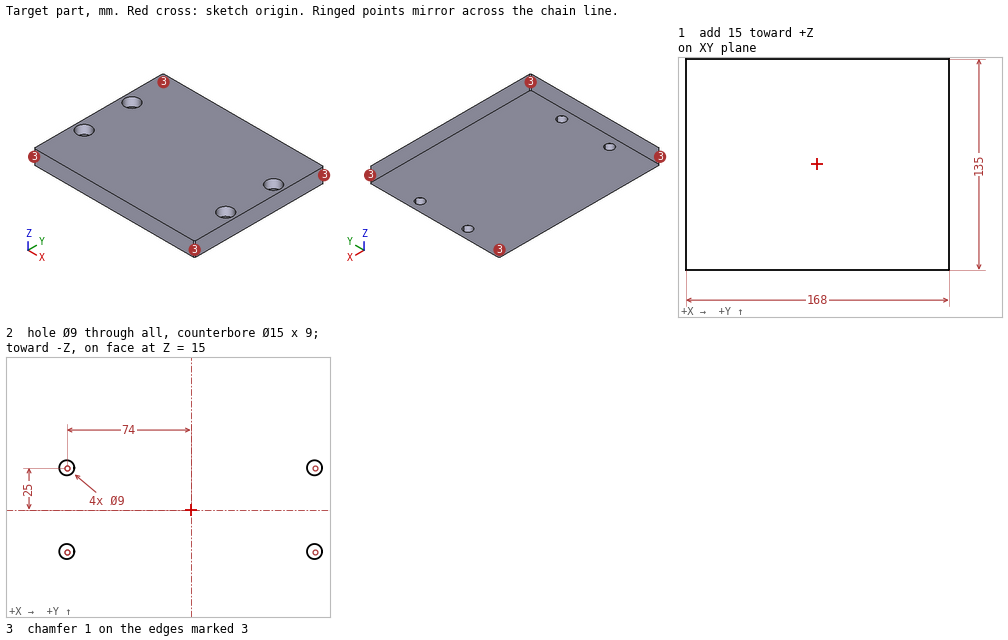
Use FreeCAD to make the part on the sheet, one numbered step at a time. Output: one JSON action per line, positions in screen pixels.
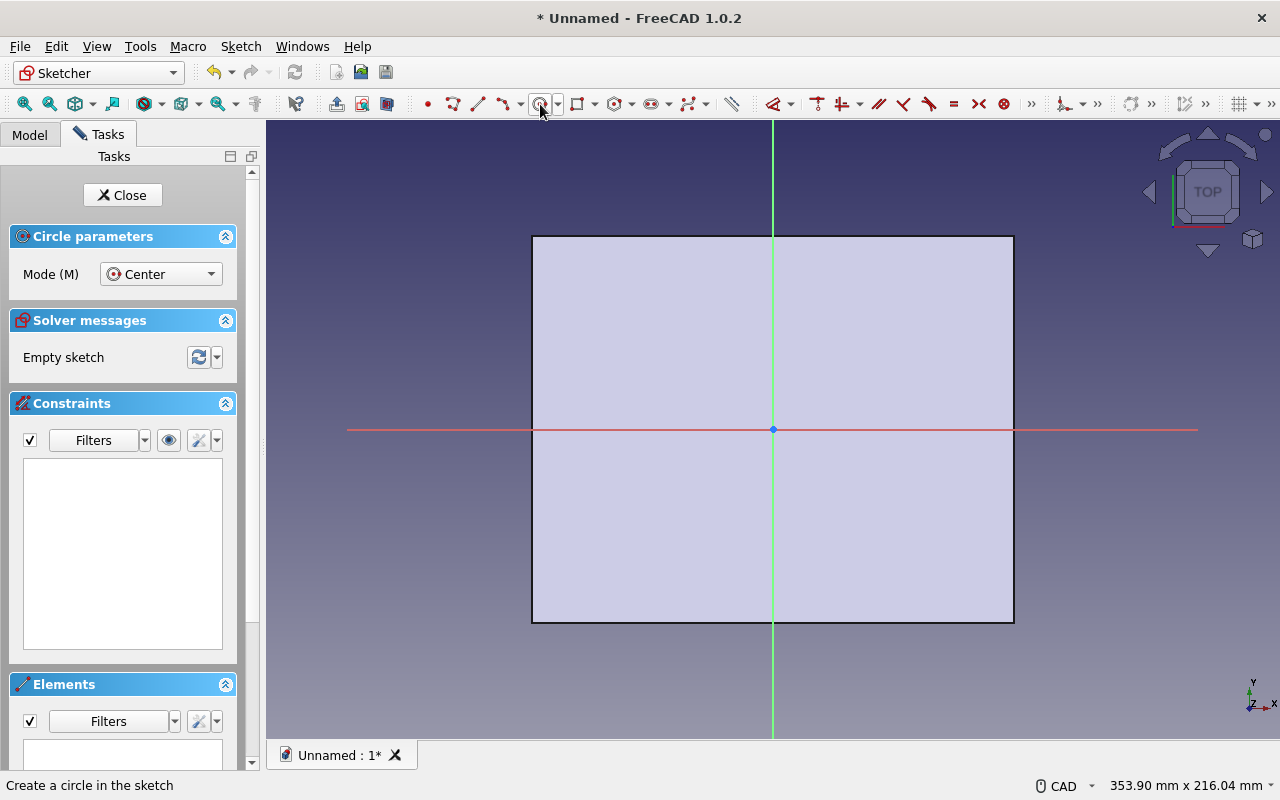
{"action": "scroll", "coordinate": [561, 358], "scroll_direction": "up", "scroll_amount": 3}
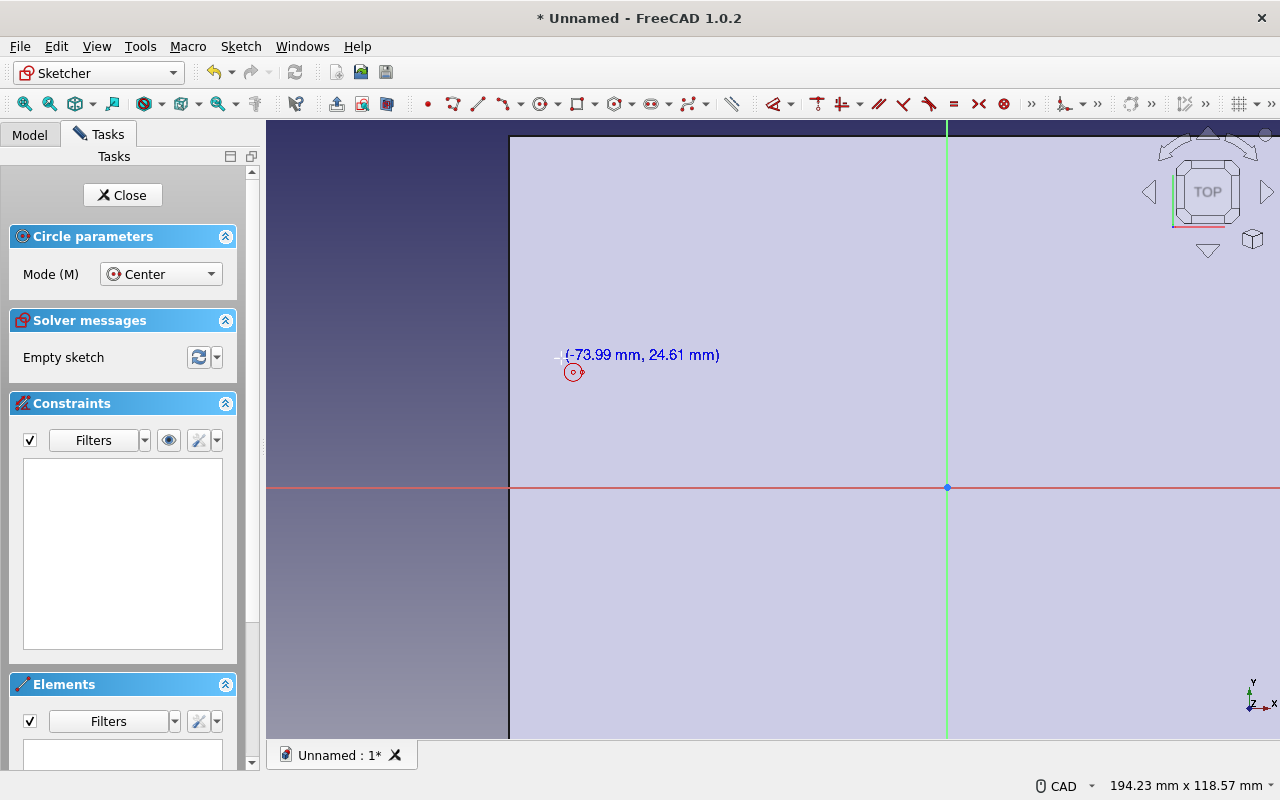
{"action": "left_click", "coordinate": [561, 357]}
{"action": "left_click", "coordinate": [577, 341]}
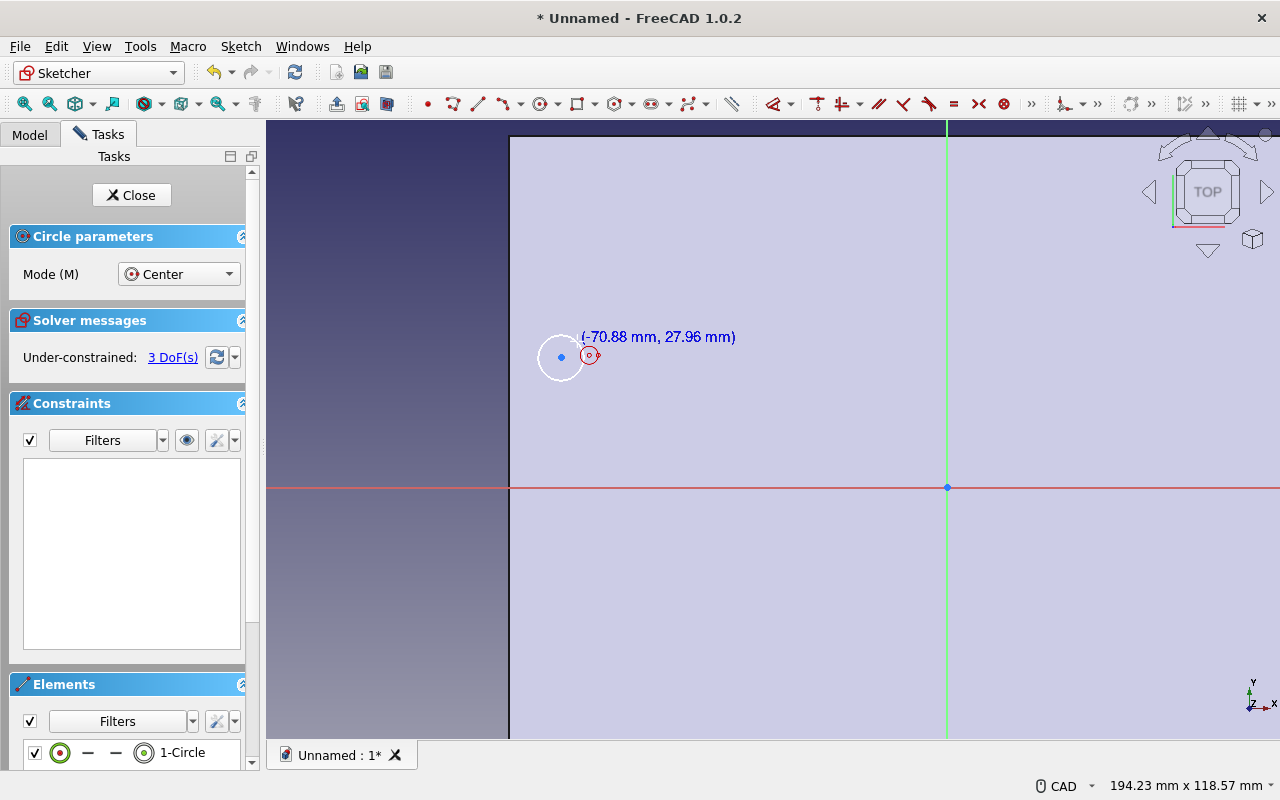
{"action": "left_click", "coordinate": [561, 618]}
{"action": "left_click", "coordinate": [577, 602]}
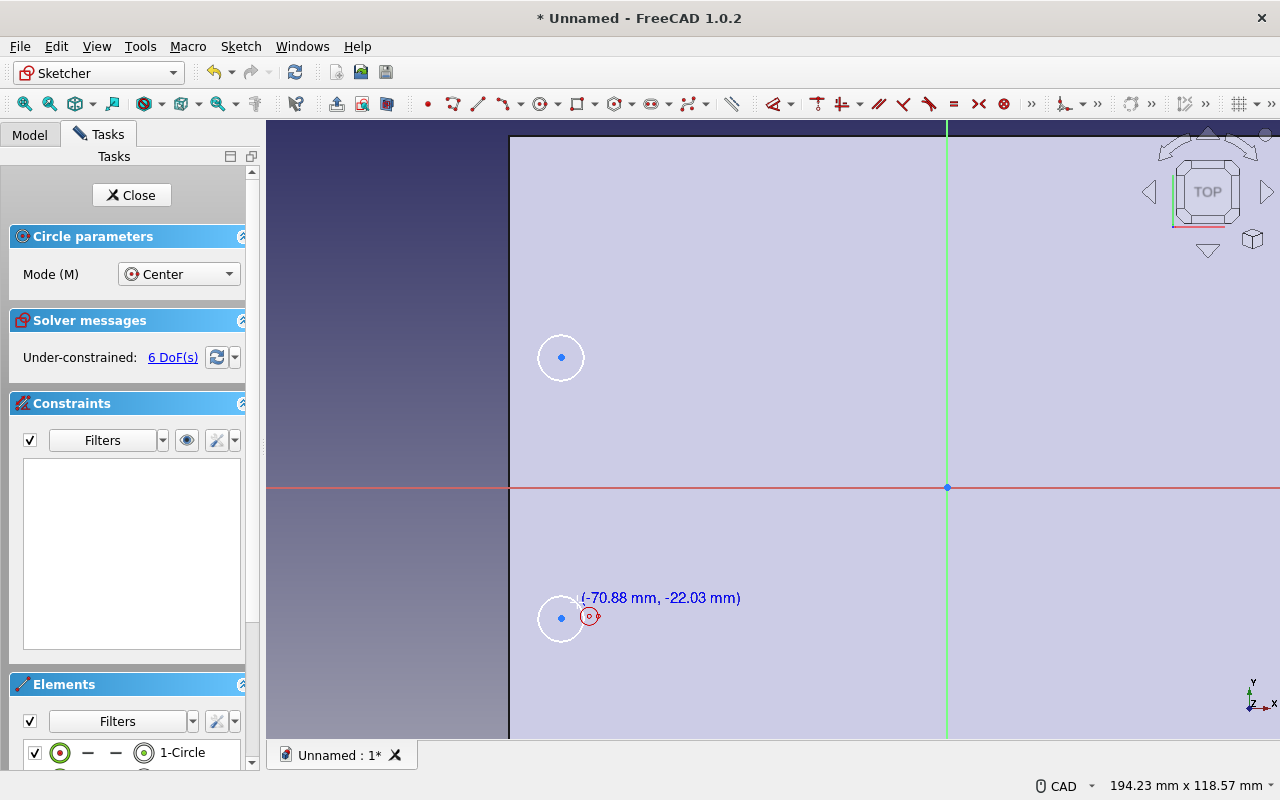
{"action": "scroll", "coordinate": [294, 311], "scroll_direction": "down", "scroll_amount": 2}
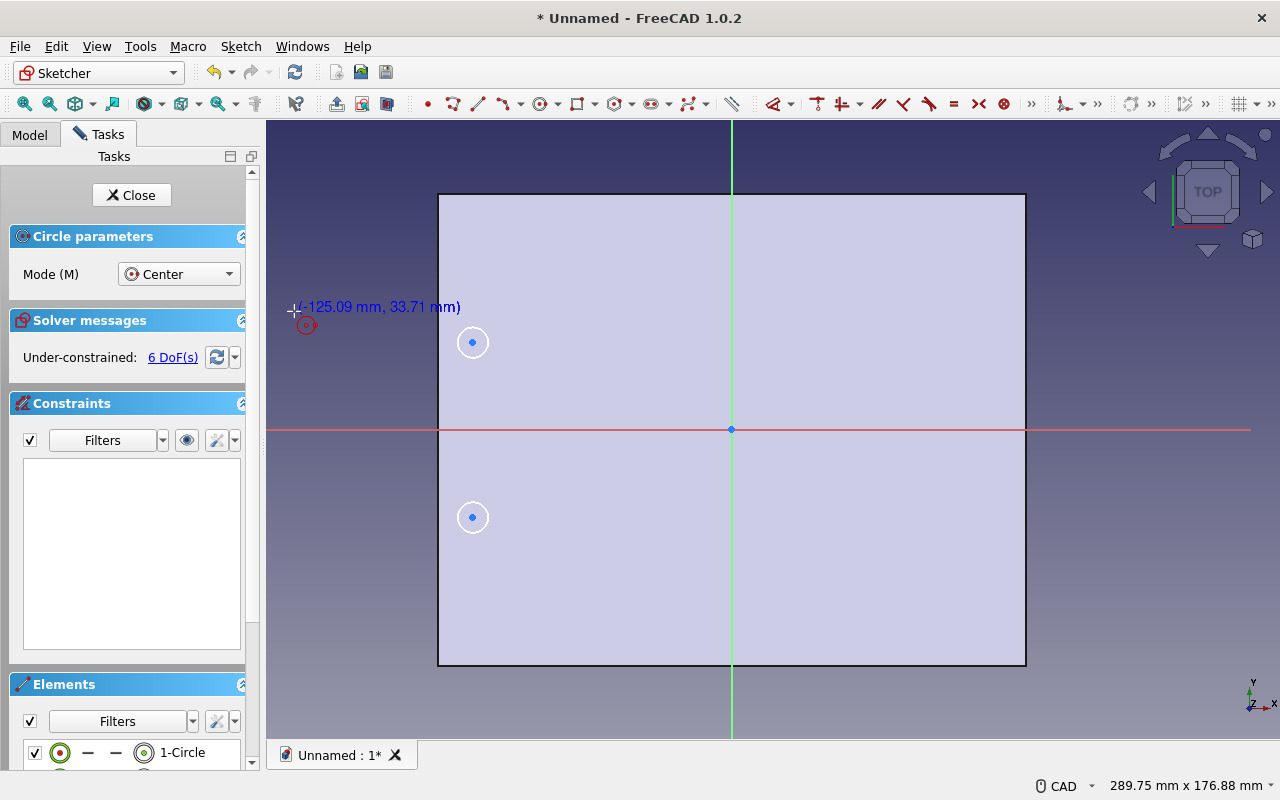
{"action": "scroll", "coordinate": [991, 517], "scroll_direction": "up", "scroll_amount": 2}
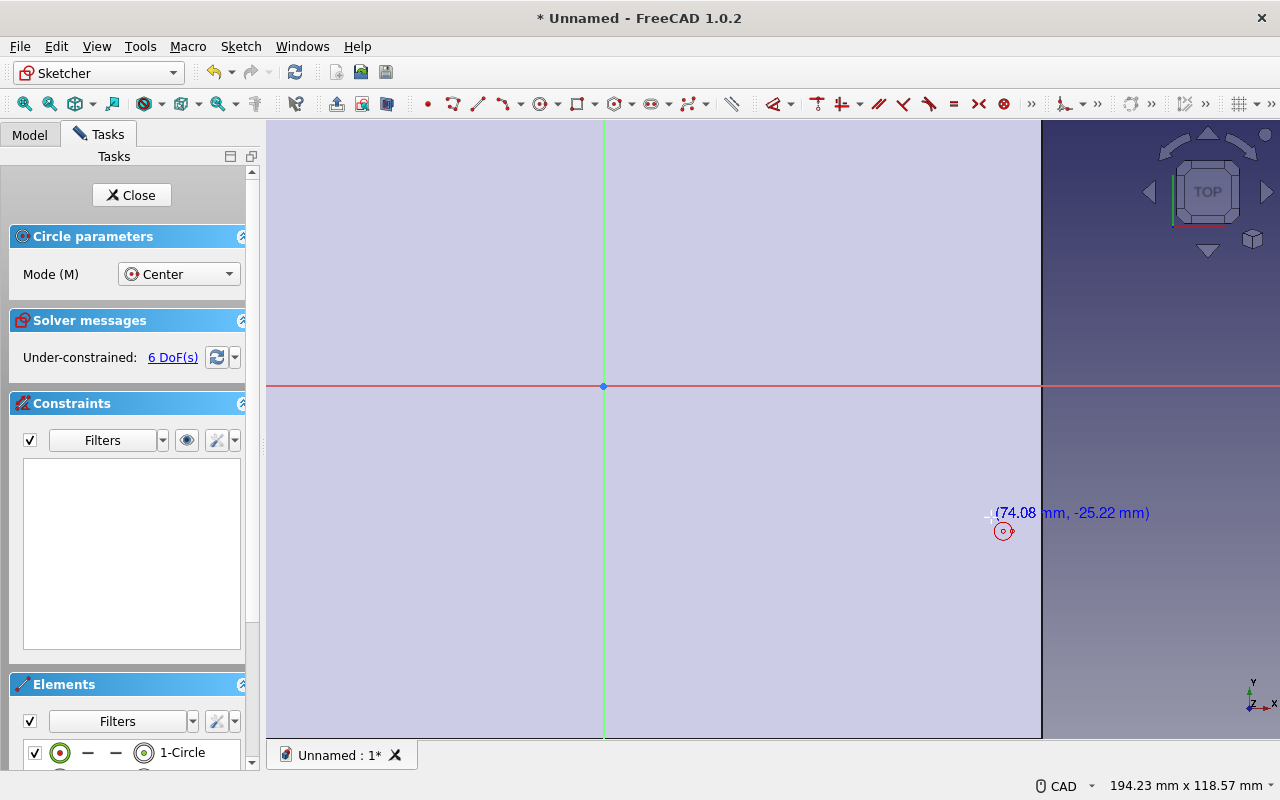
{"action": "left_click", "coordinate": [990, 517]}
{"action": "left_click", "coordinate": [1007, 500]}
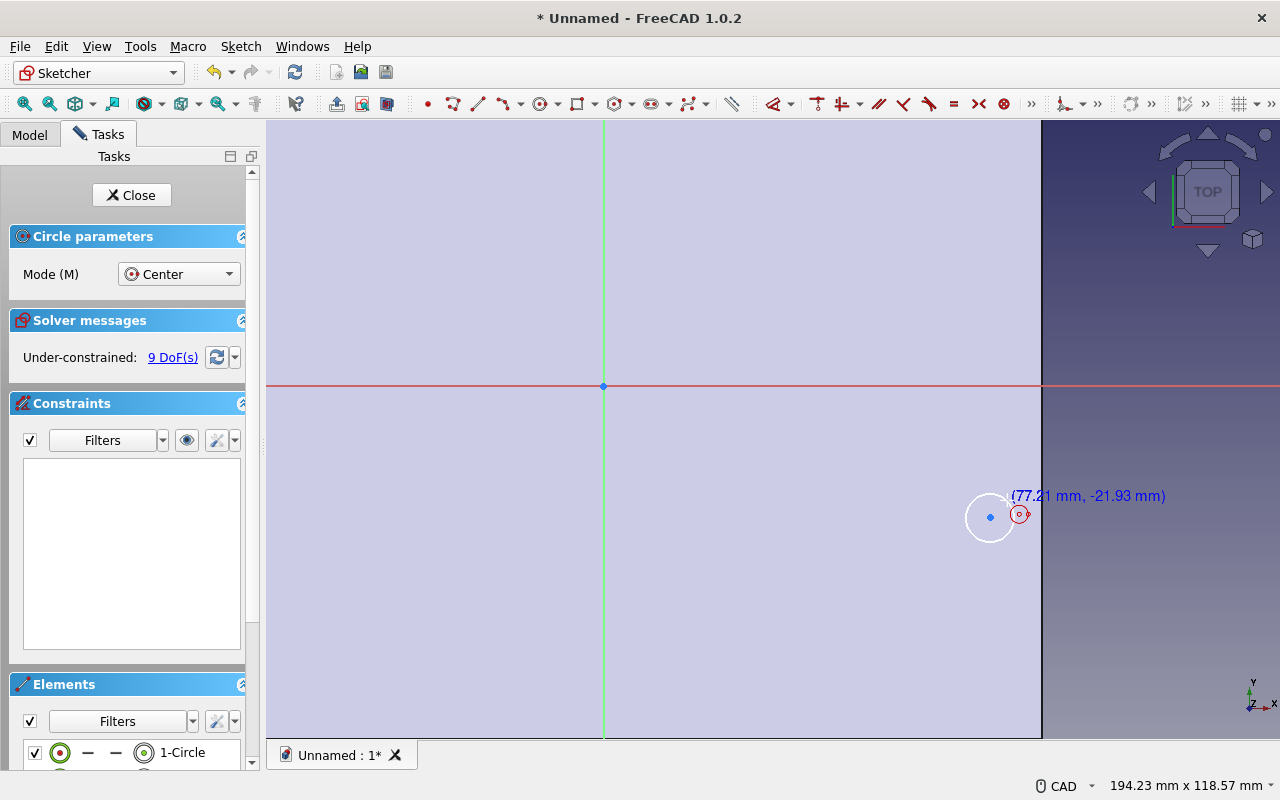
{"action": "left_click", "coordinate": [990, 256]}
{"action": "left_click", "coordinate": [1007, 239]}
{"action": "key", "text": "Escape"}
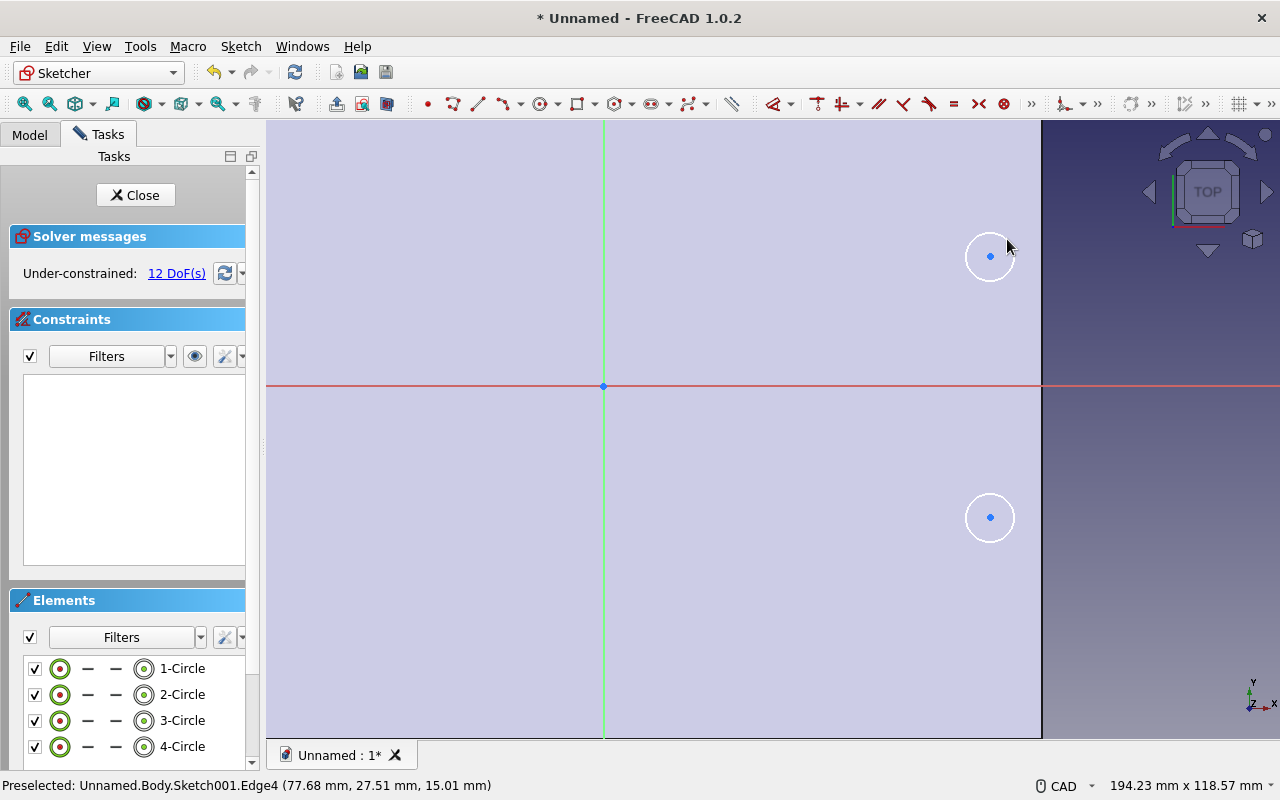
{"action": "scroll", "coordinate": [909, 517], "scroll_direction": "down", "scroll_amount": 2}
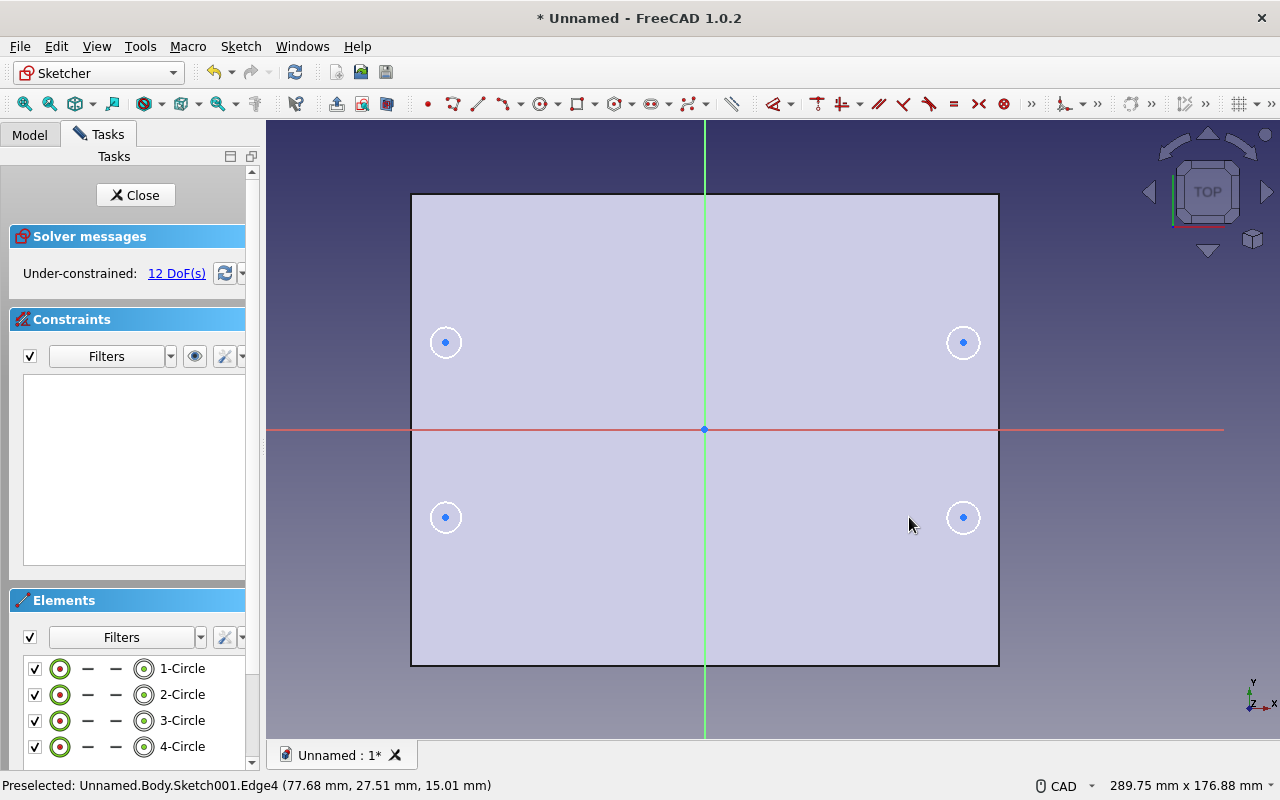
{"action": "left_click", "coordinate": [457, 332]}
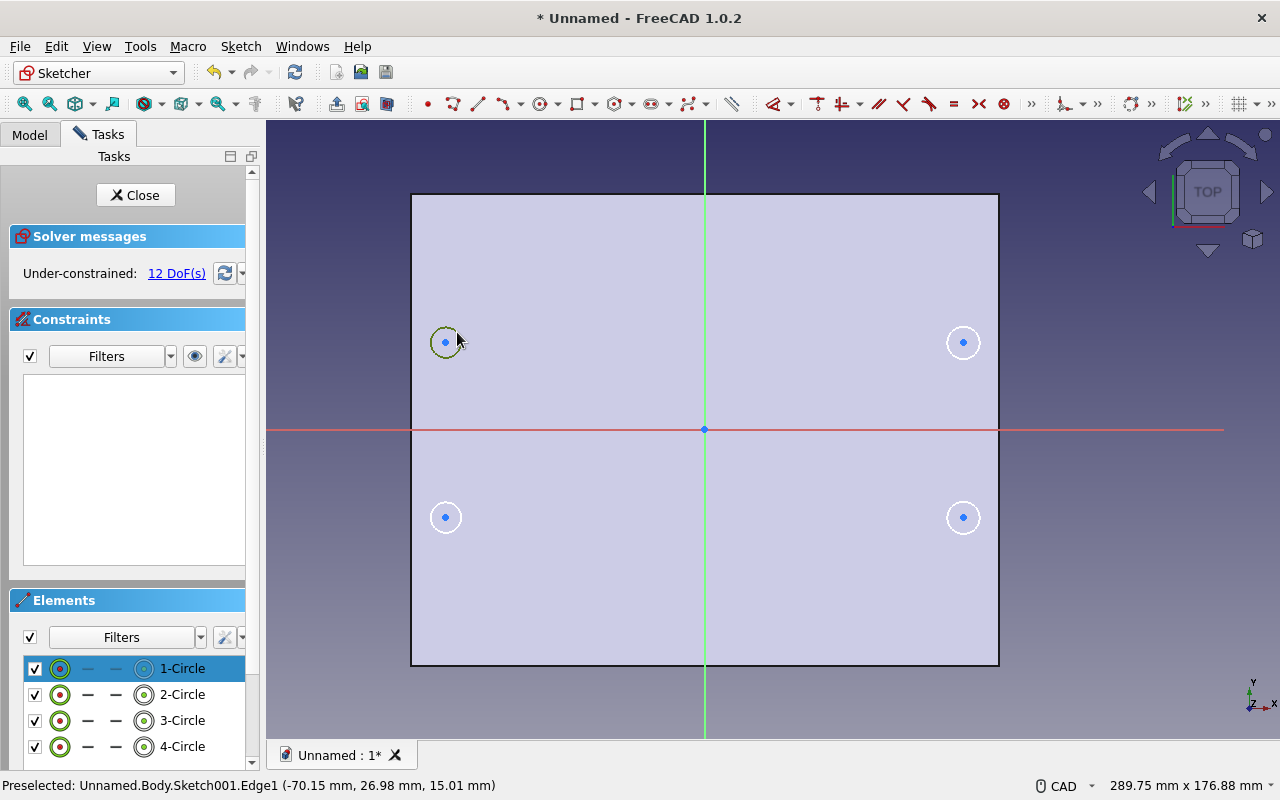
{"action": "left_click", "coordinate": [457, 507]}